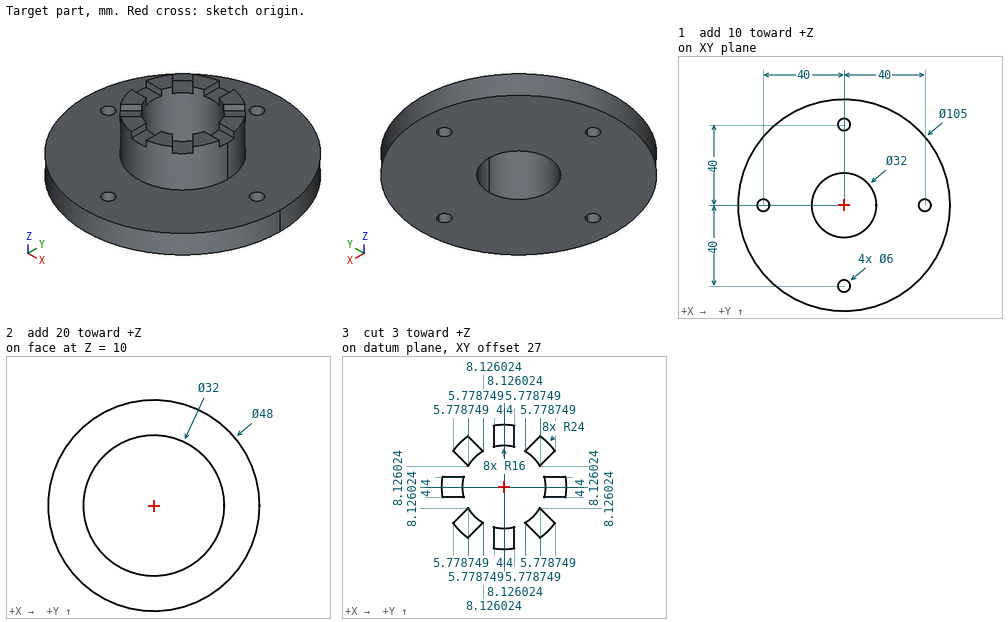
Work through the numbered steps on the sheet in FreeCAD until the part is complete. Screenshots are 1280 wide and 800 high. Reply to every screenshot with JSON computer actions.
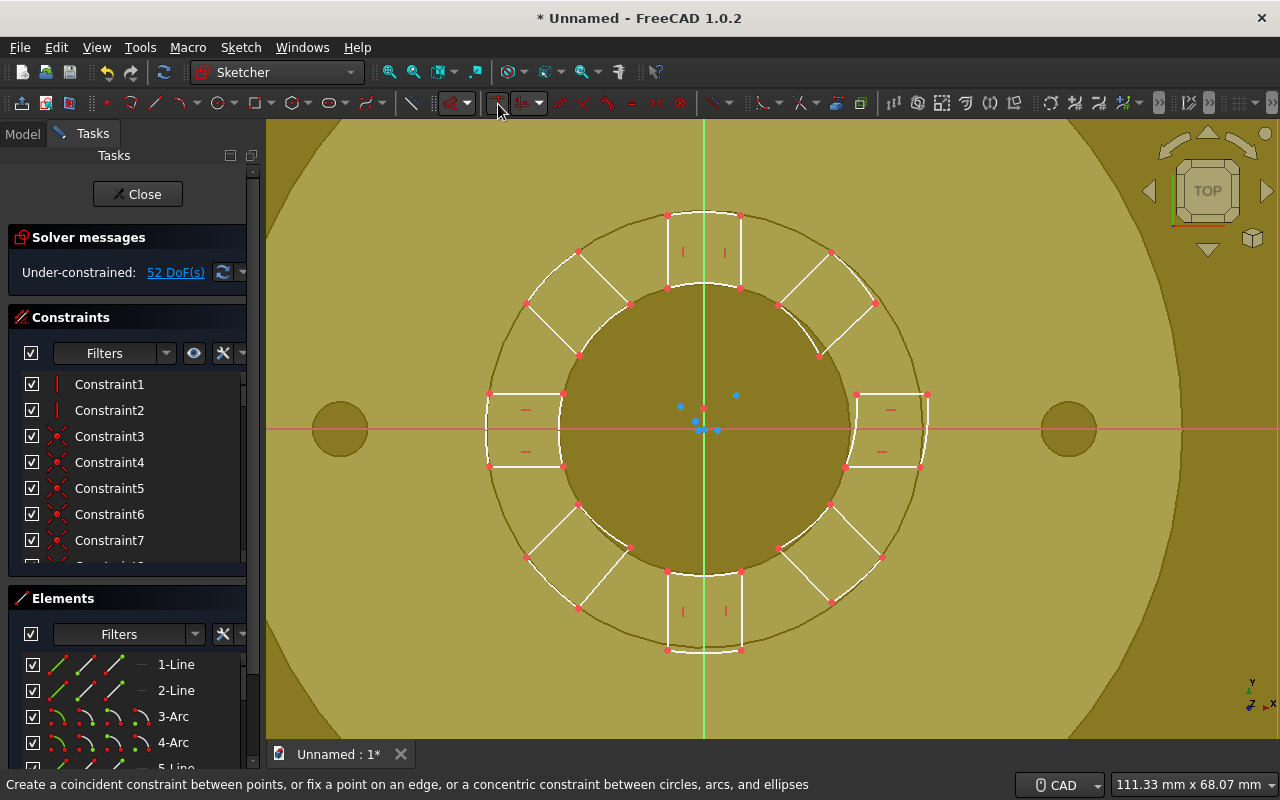
{"action": "left_click", "coordinate": [719, 284]}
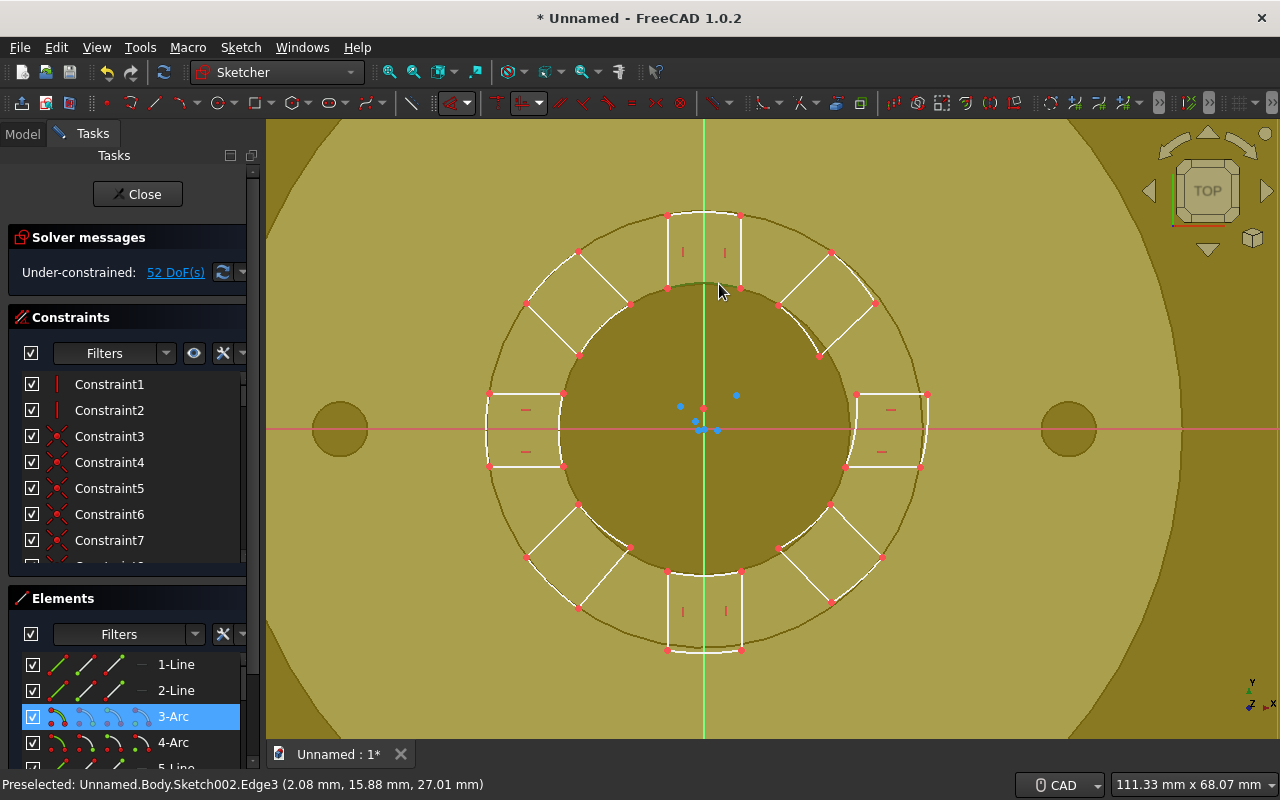
{"action": "left_click", "coordinate": [540, 574]}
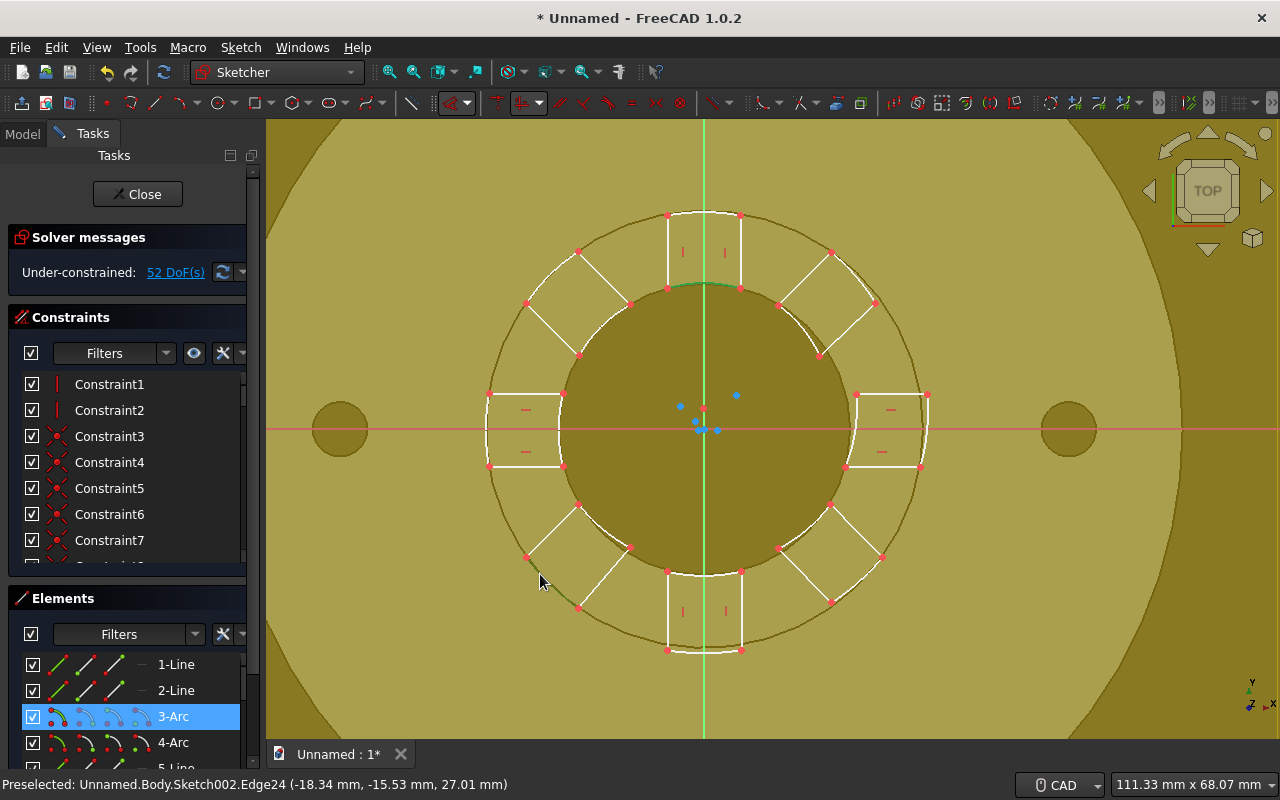
{"action": "left_click", "coordinate": [498, 104]}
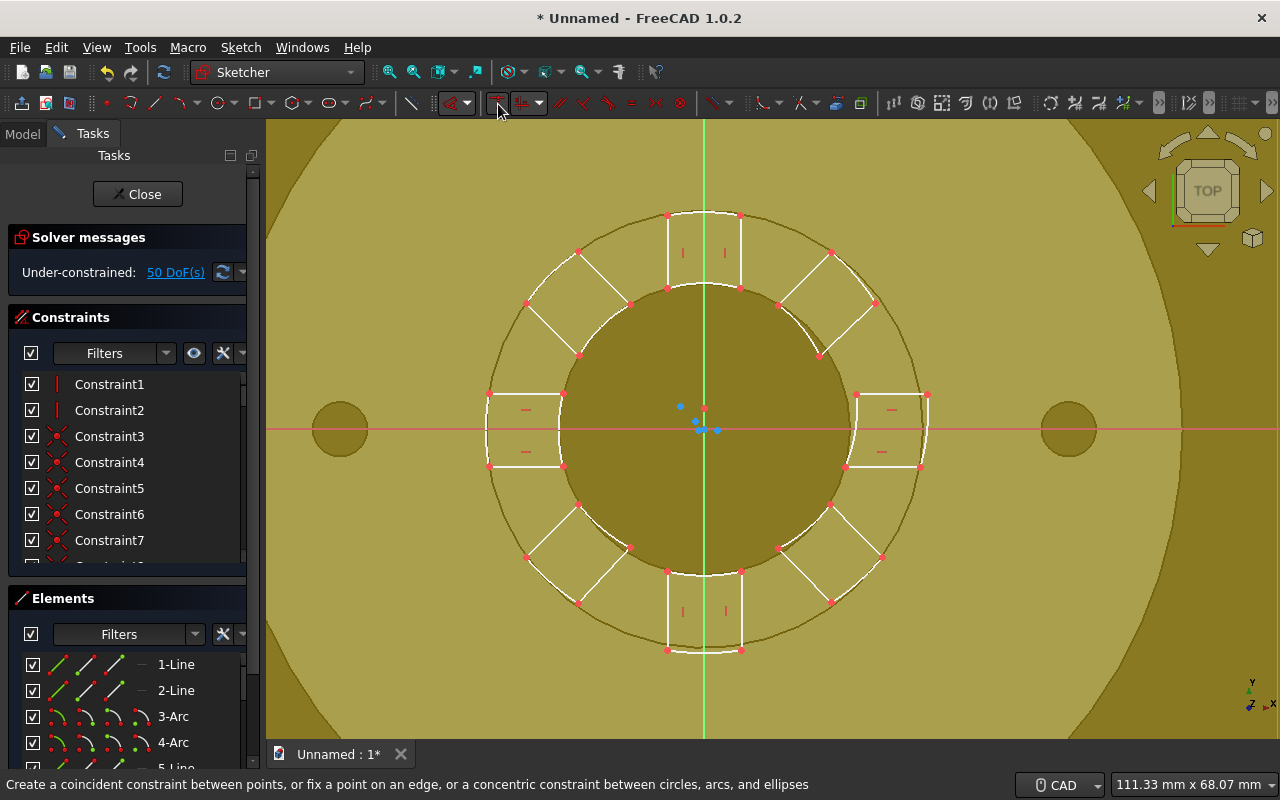
{"action": "left_click", "coordinate": [719, 284]}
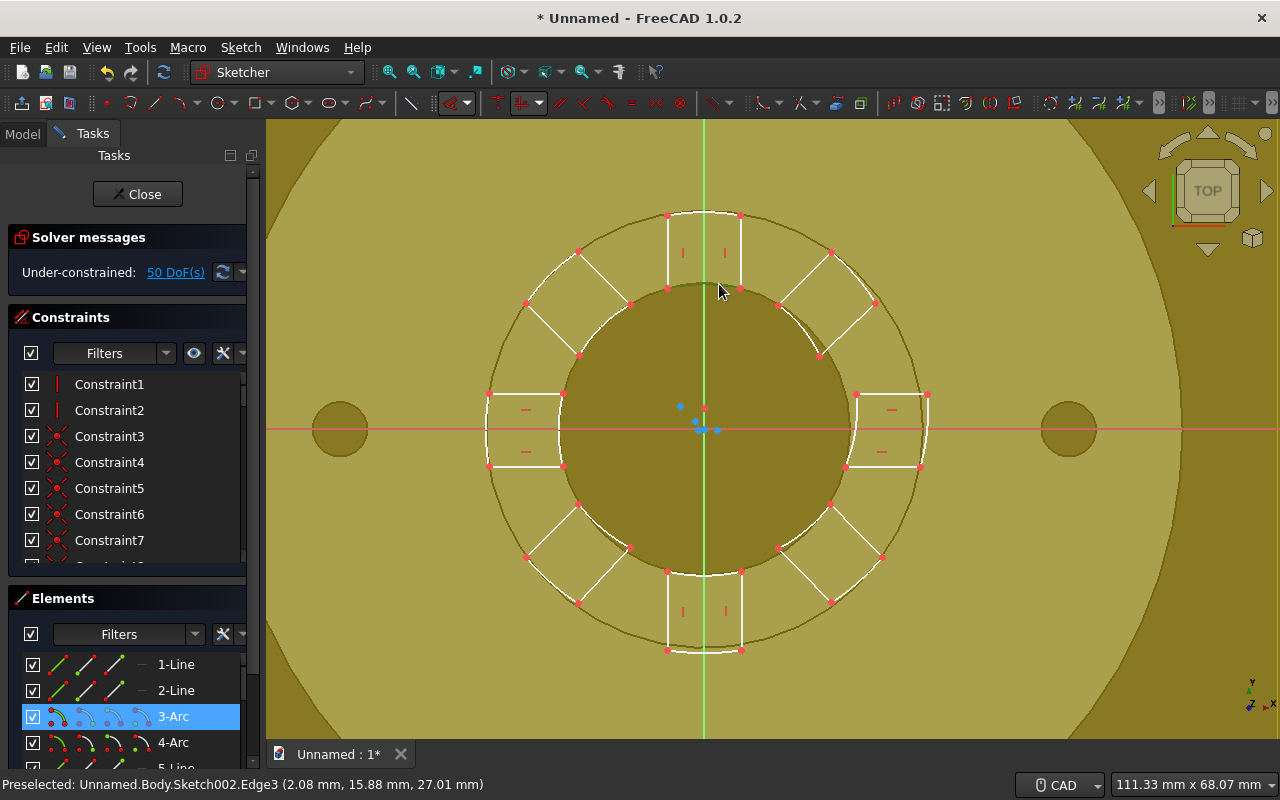
{"action": "left_click", "coordinate": [559, 416]}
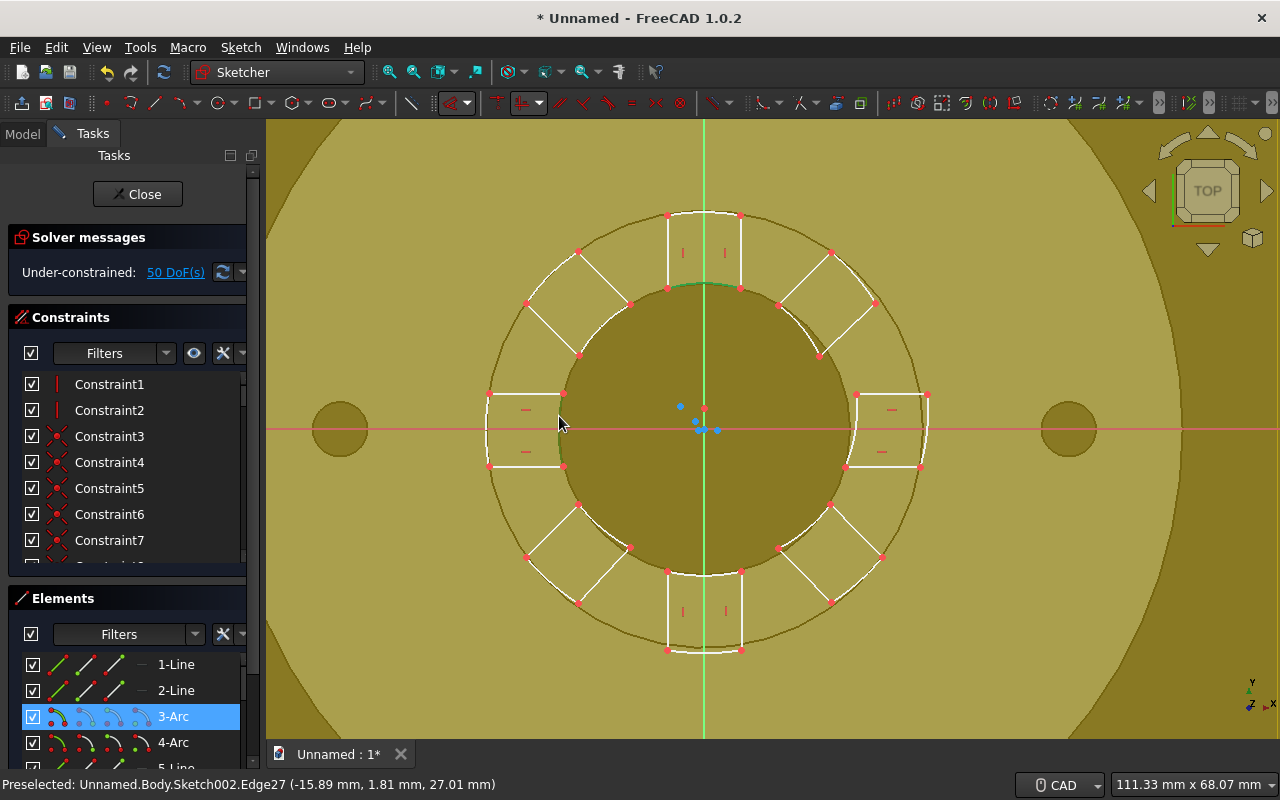
{"action": "left_click", "coordinate": [498, 104]}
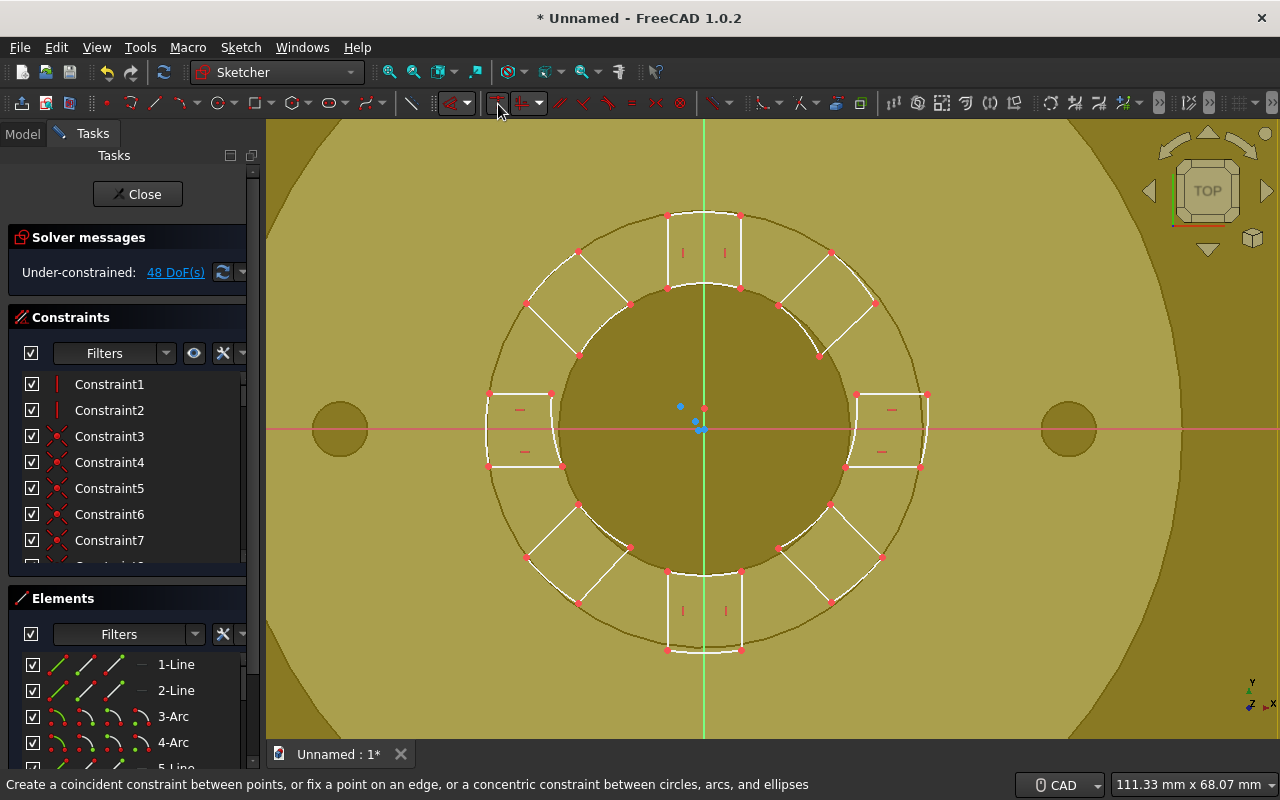
{"action": "left_click", "coordinate": [719, 284]}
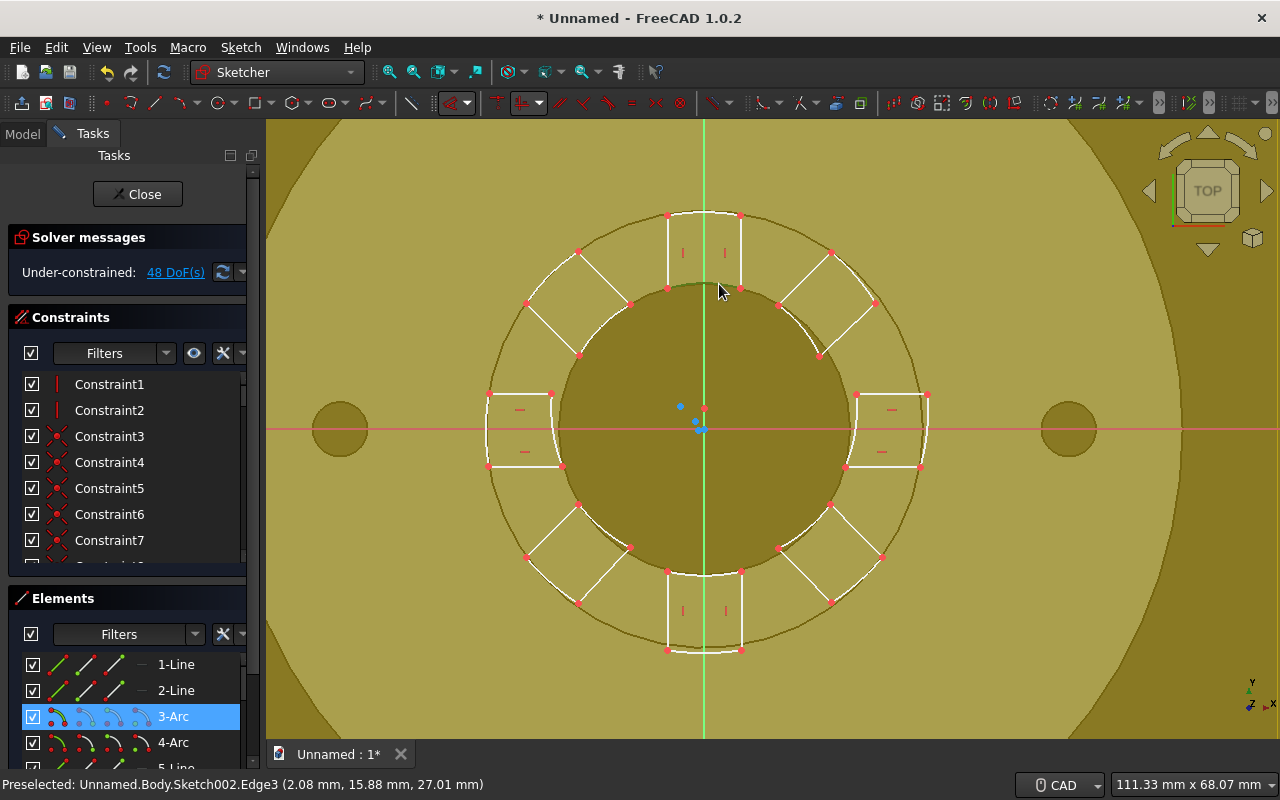
{"action": "left_click", "coordinate": [486, 416]}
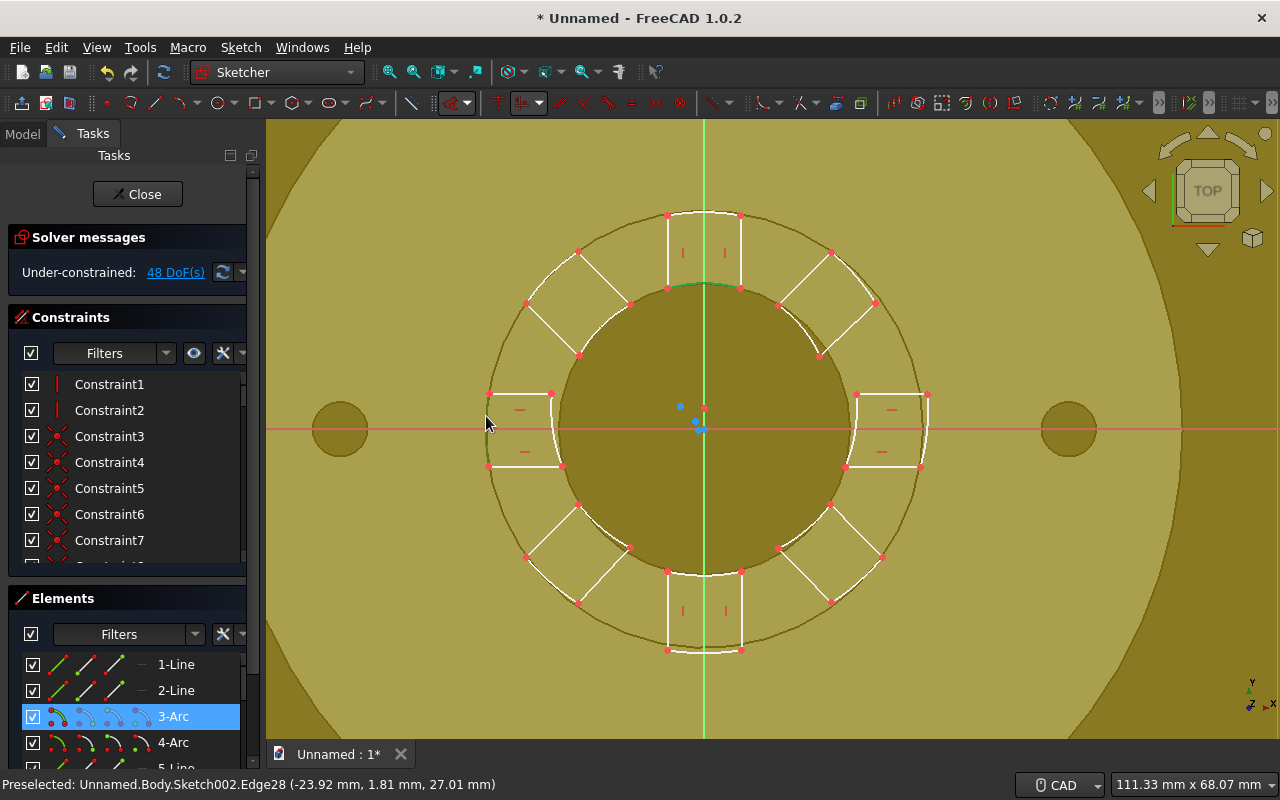
{"action": "left_click", "coordinate": [498, 104]}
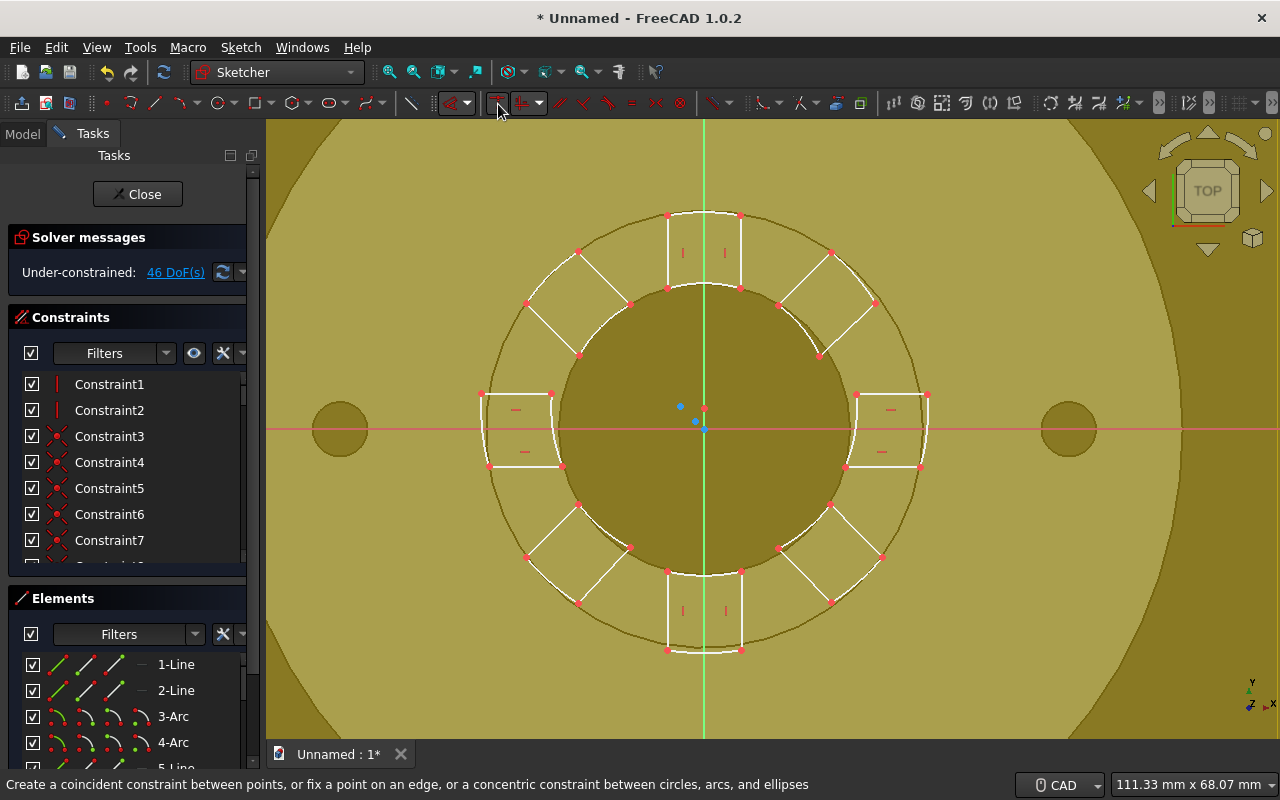
{"action": "left_click", "coordinate": [719, 284]}